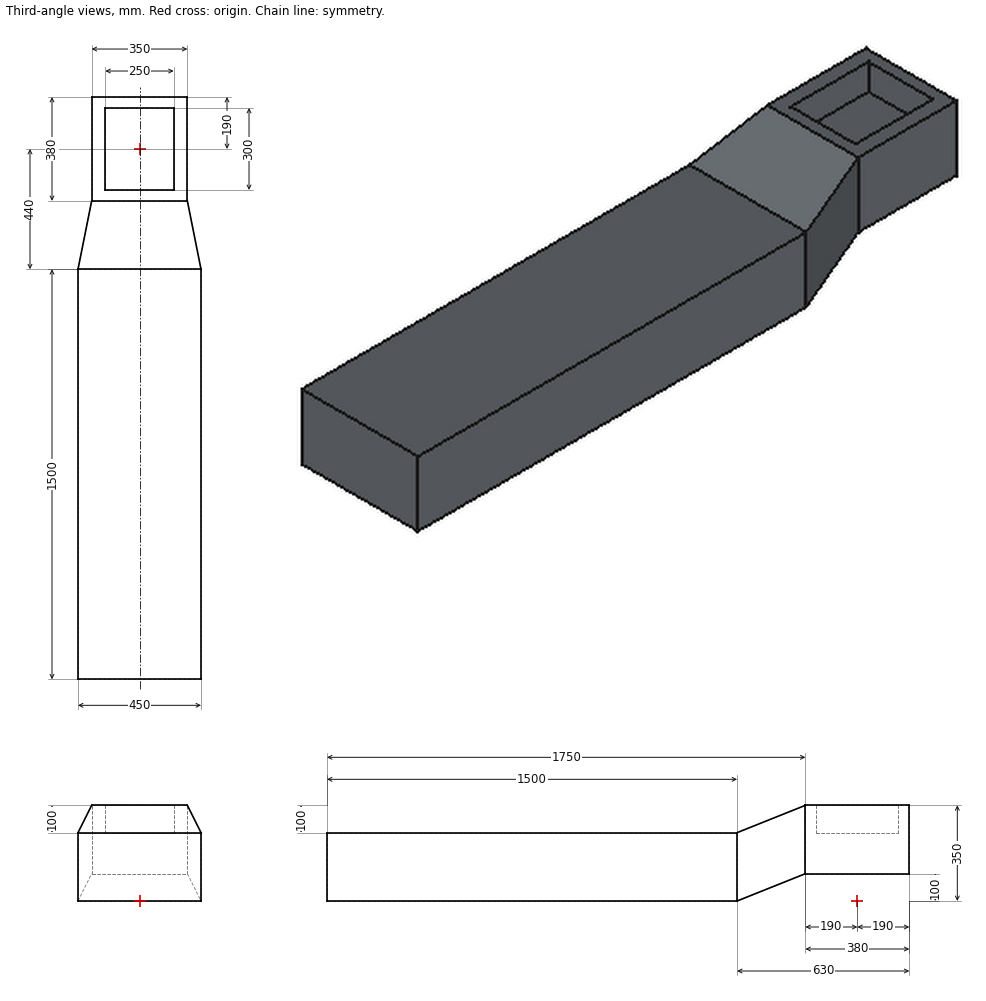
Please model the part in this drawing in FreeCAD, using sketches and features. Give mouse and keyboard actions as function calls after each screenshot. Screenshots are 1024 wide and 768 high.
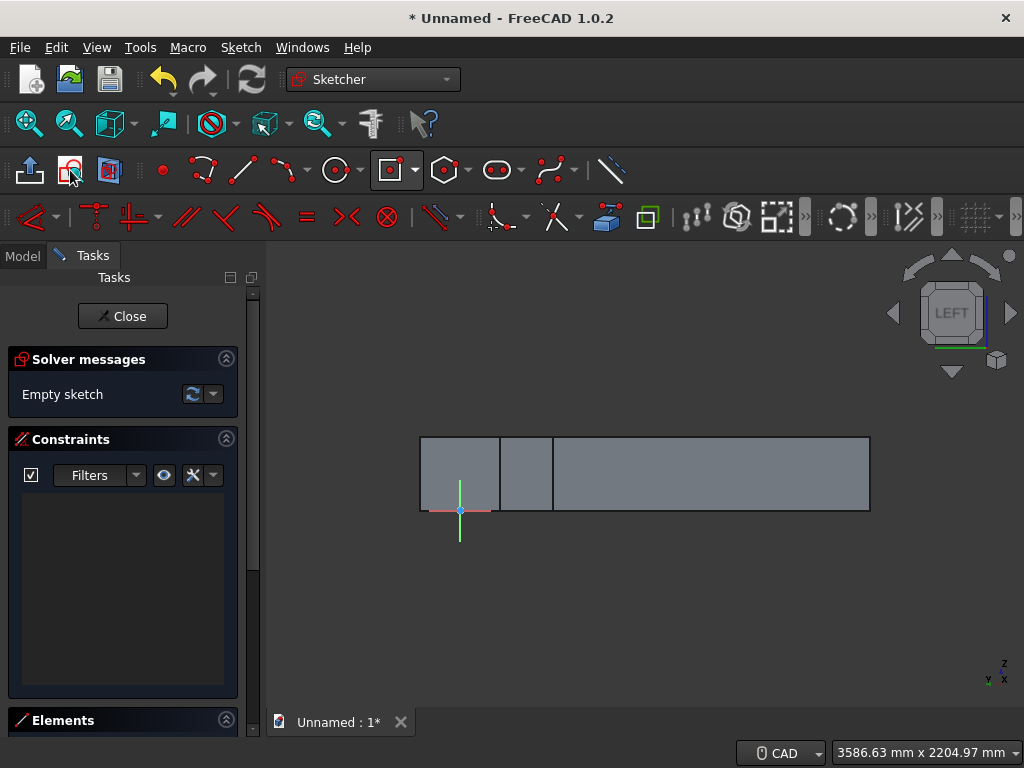
scroll(294, 474, down, 1)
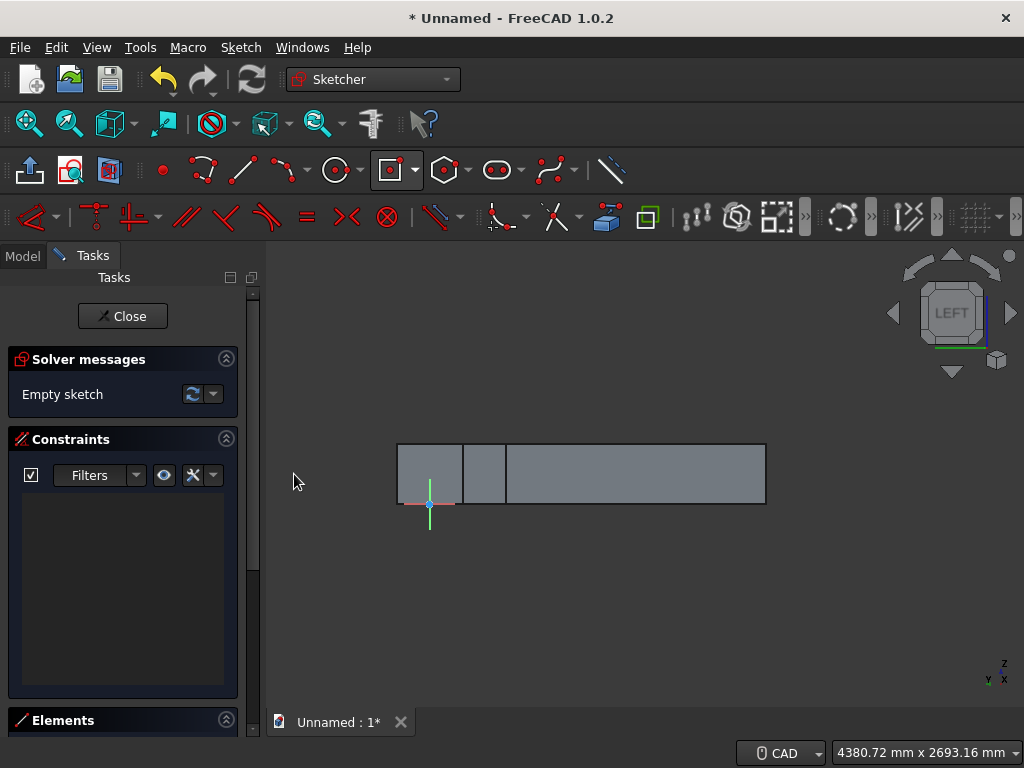
click(204, 170)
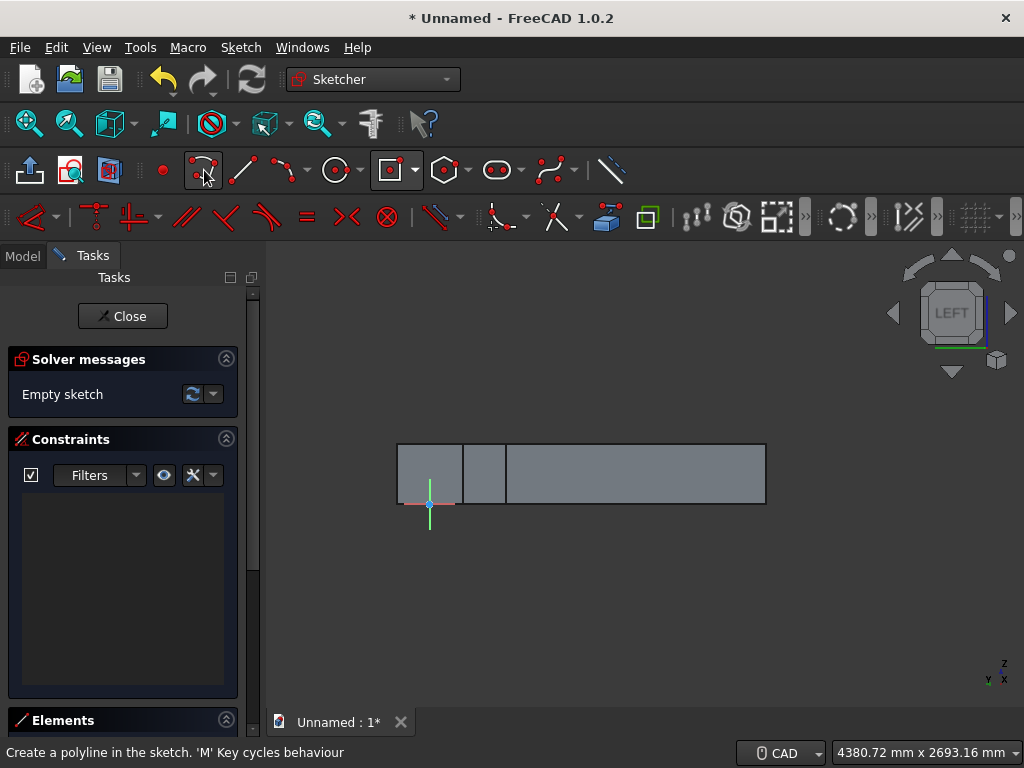
click(463, 444)
click(506, 461)
click(766, 461)
click(766, 444)
click(463, 445)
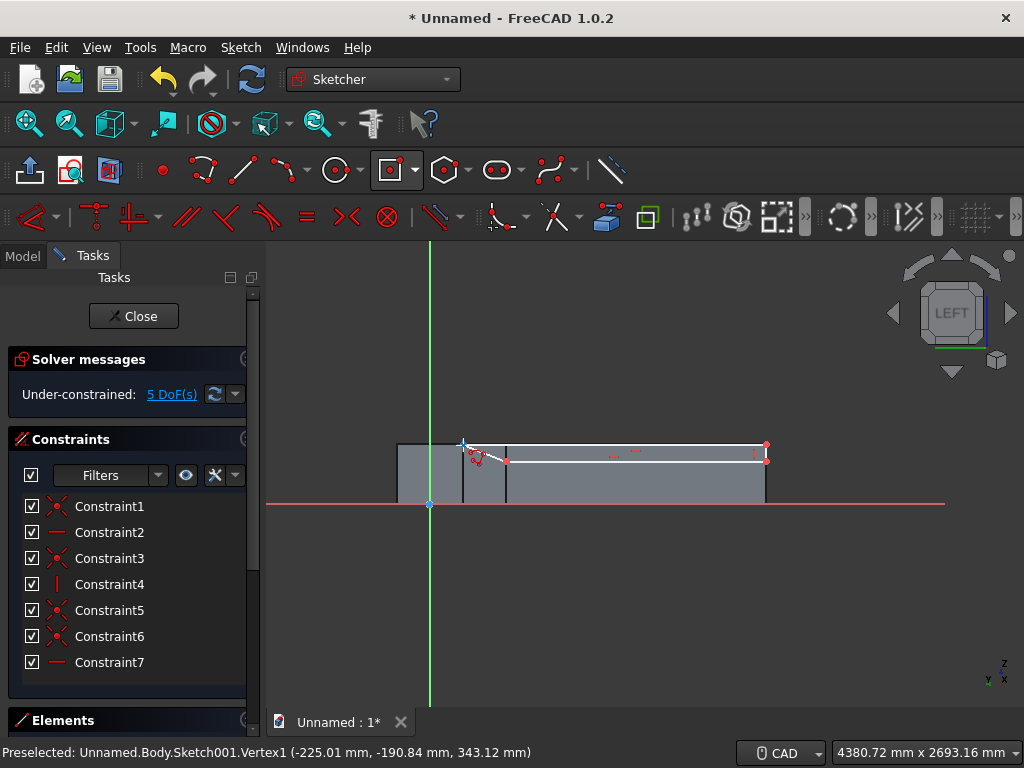
click(397, 504)
click(506, 495)
click(463, 487)
click(397, 487)
click(397, 504)
key(Escape)
key(Escape)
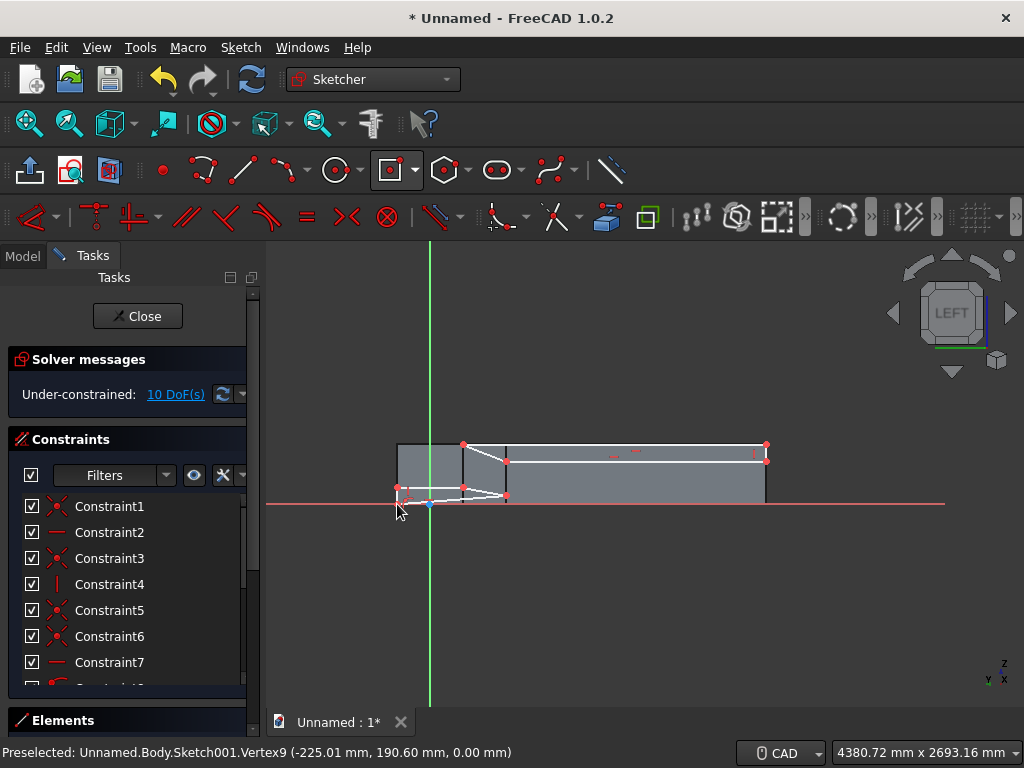
click(441, 501)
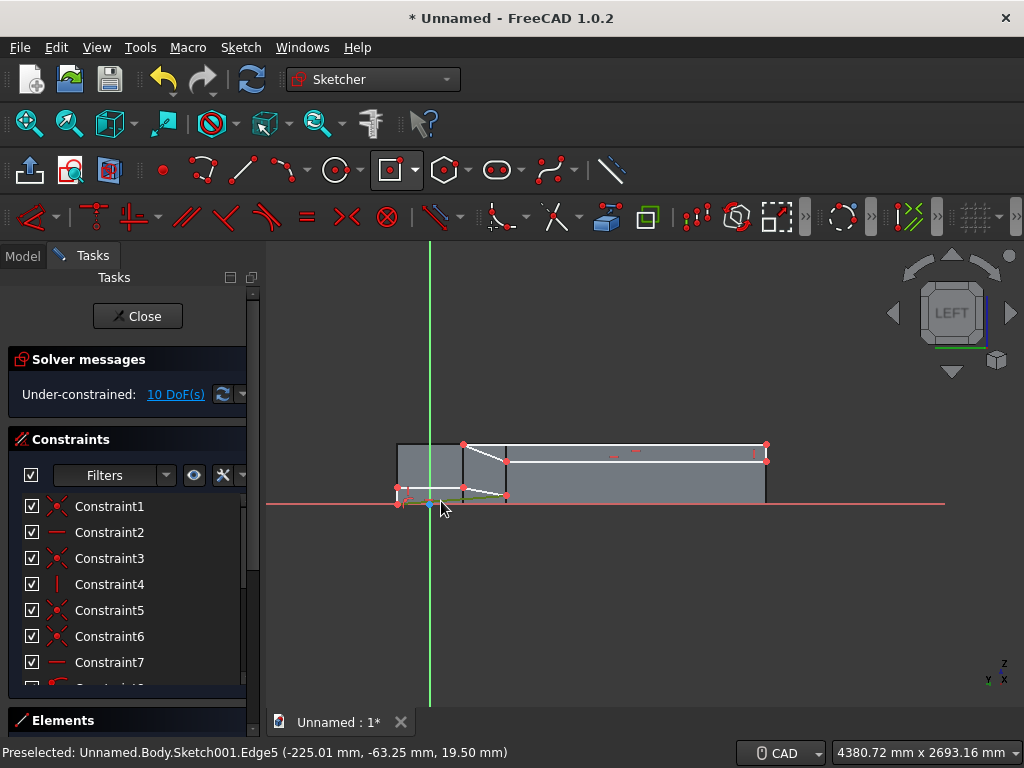
click(160, 218)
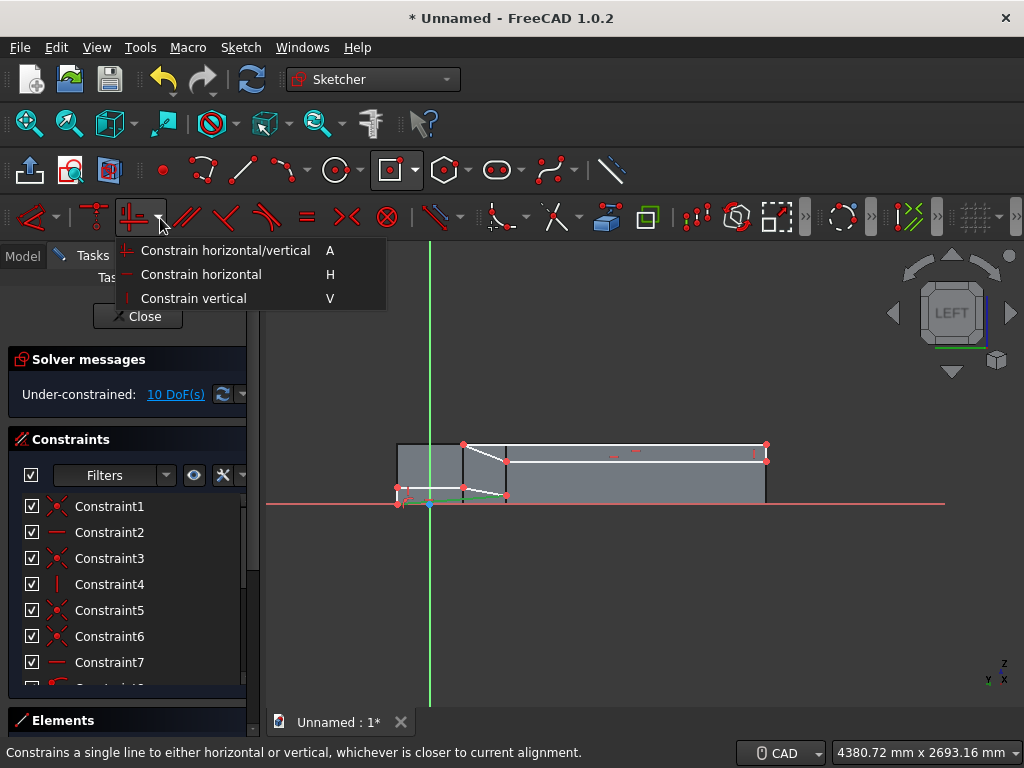
click(251, 274)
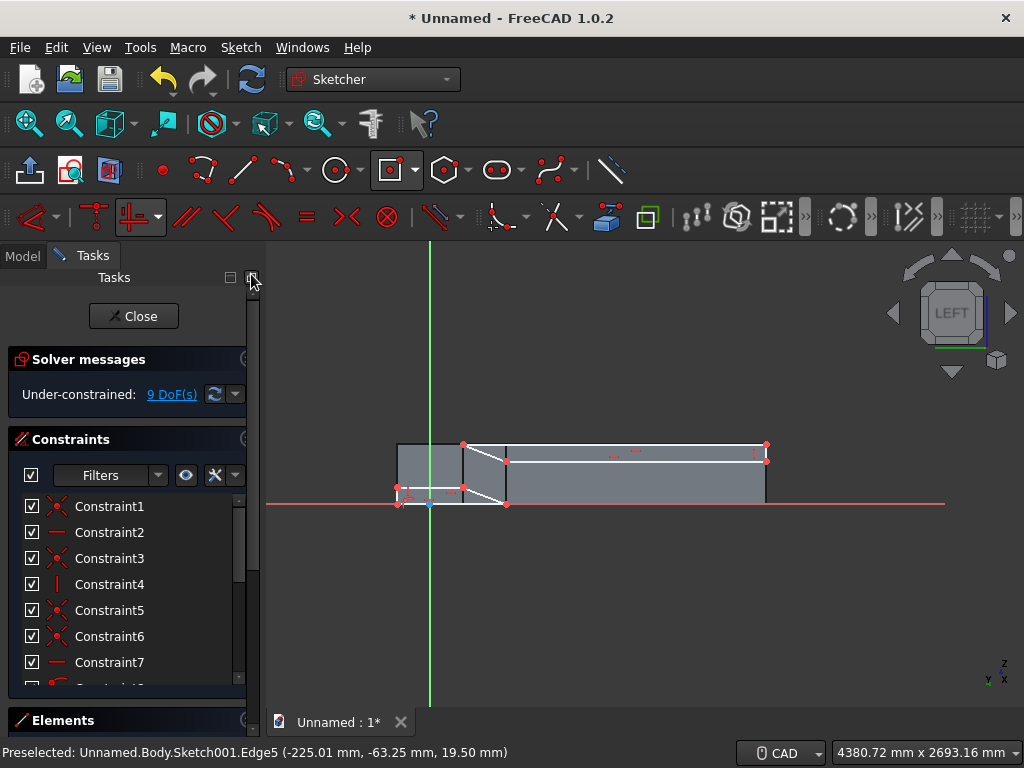
click(32, 218)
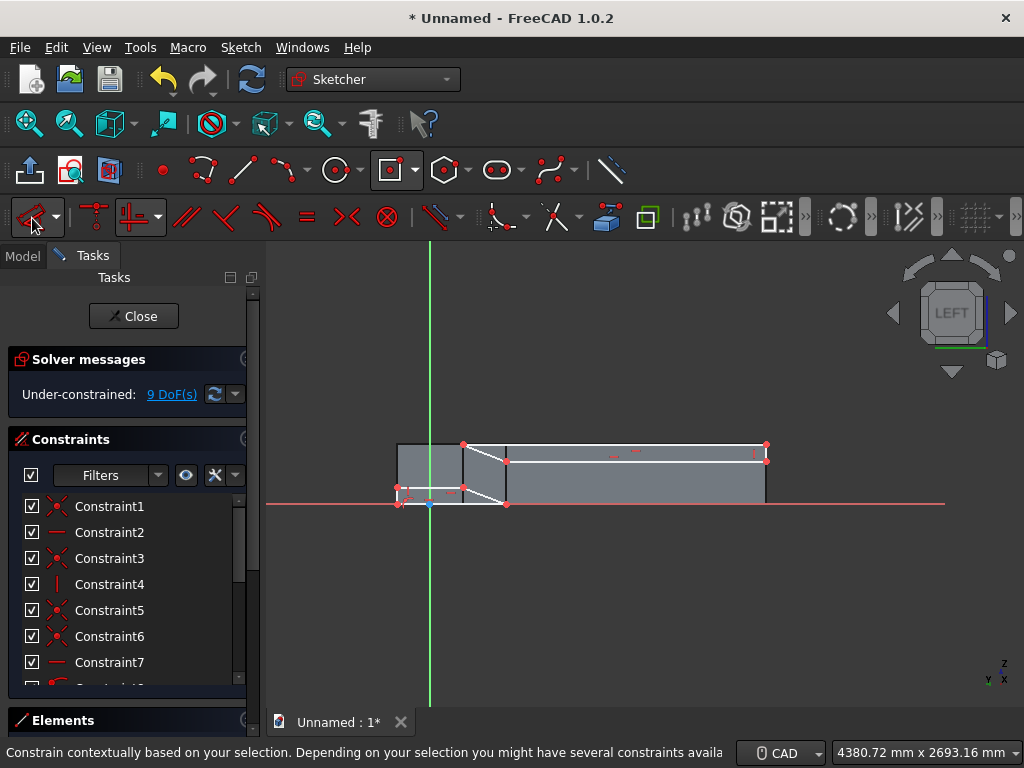
scroll(766, 454, up, 5)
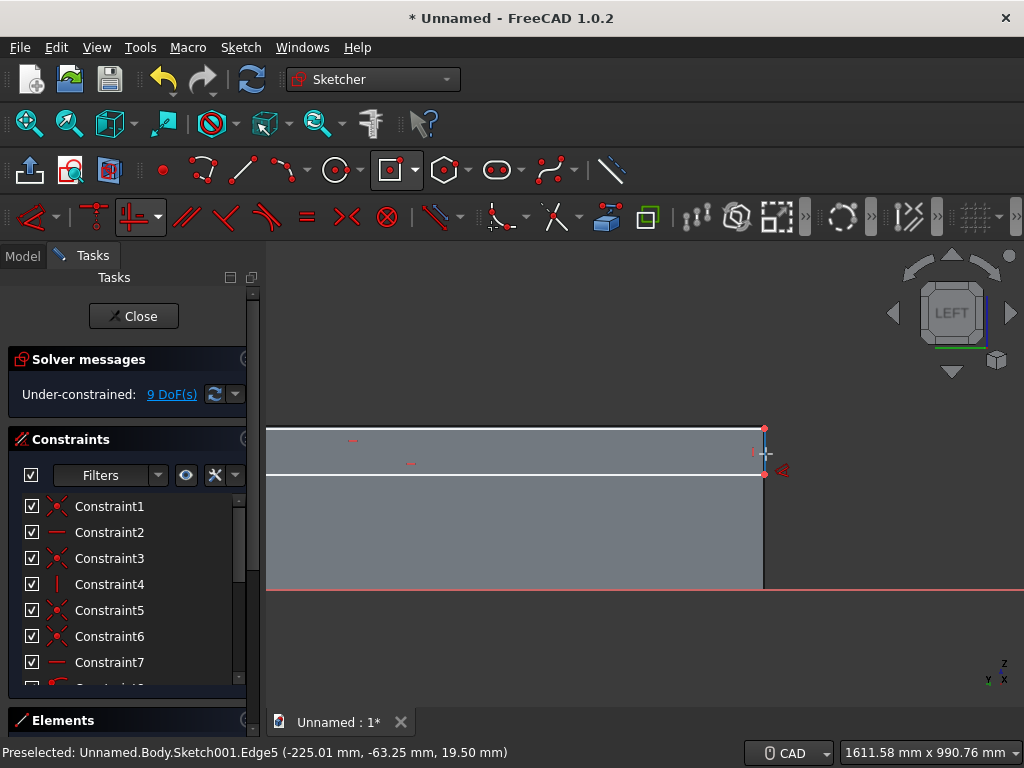
click(765, 452)
click(799, 452)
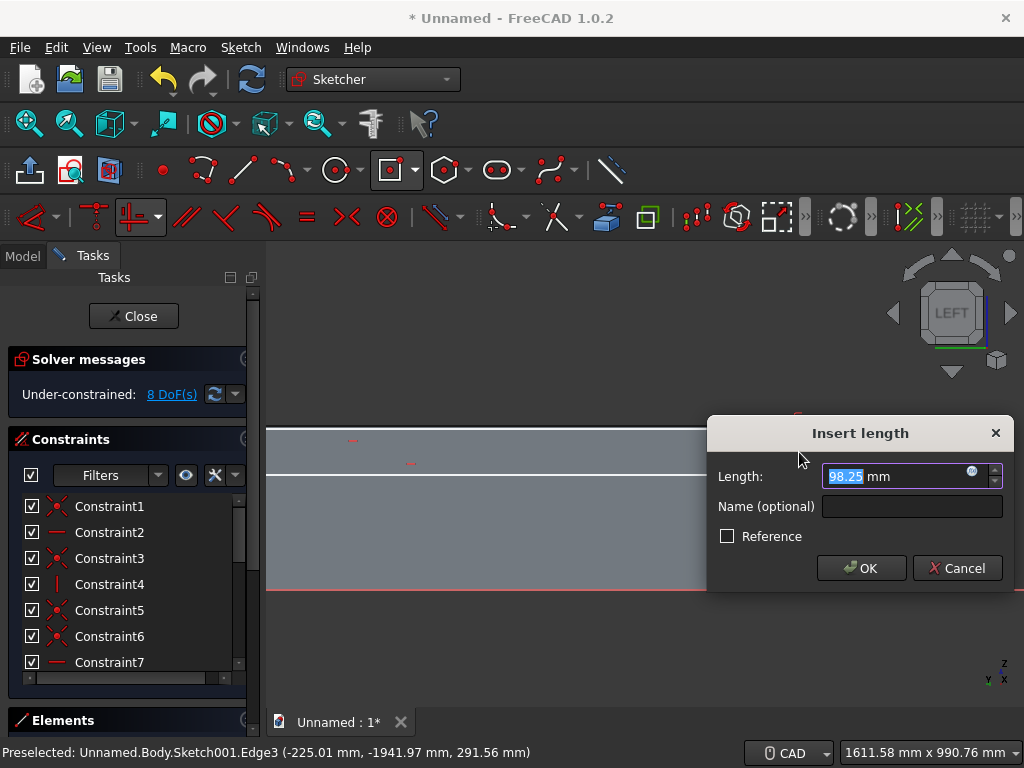
text(100)
key(Return)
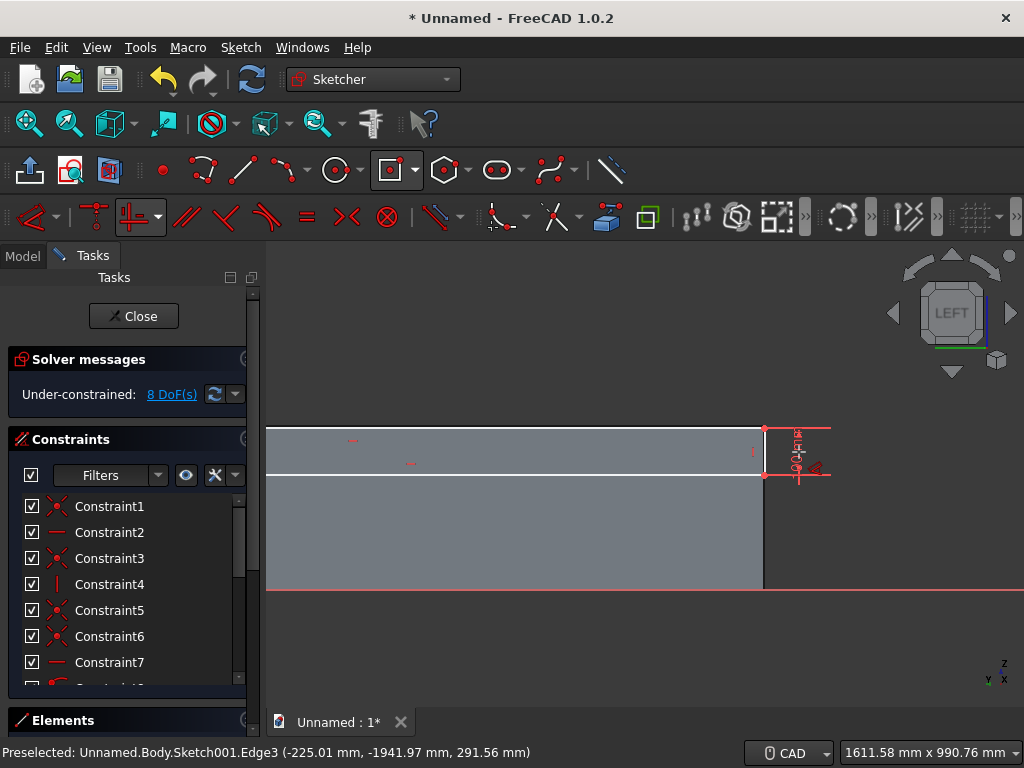
scroll(759, 454, down, 5)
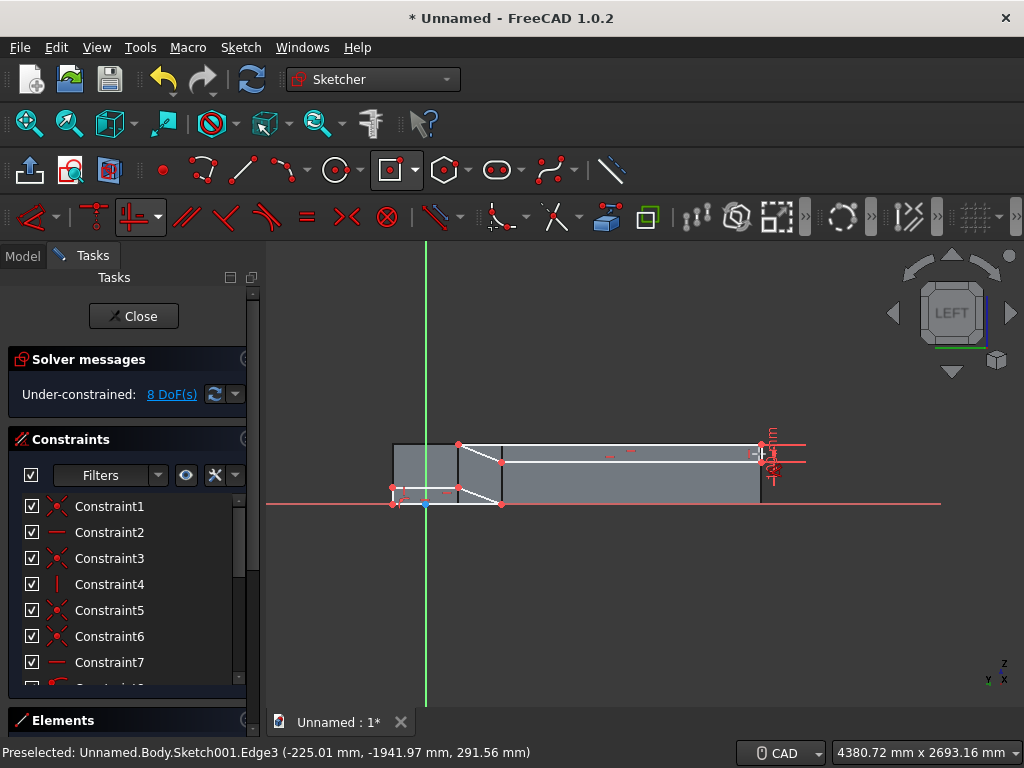
click(469, 504)
click(447, 538)